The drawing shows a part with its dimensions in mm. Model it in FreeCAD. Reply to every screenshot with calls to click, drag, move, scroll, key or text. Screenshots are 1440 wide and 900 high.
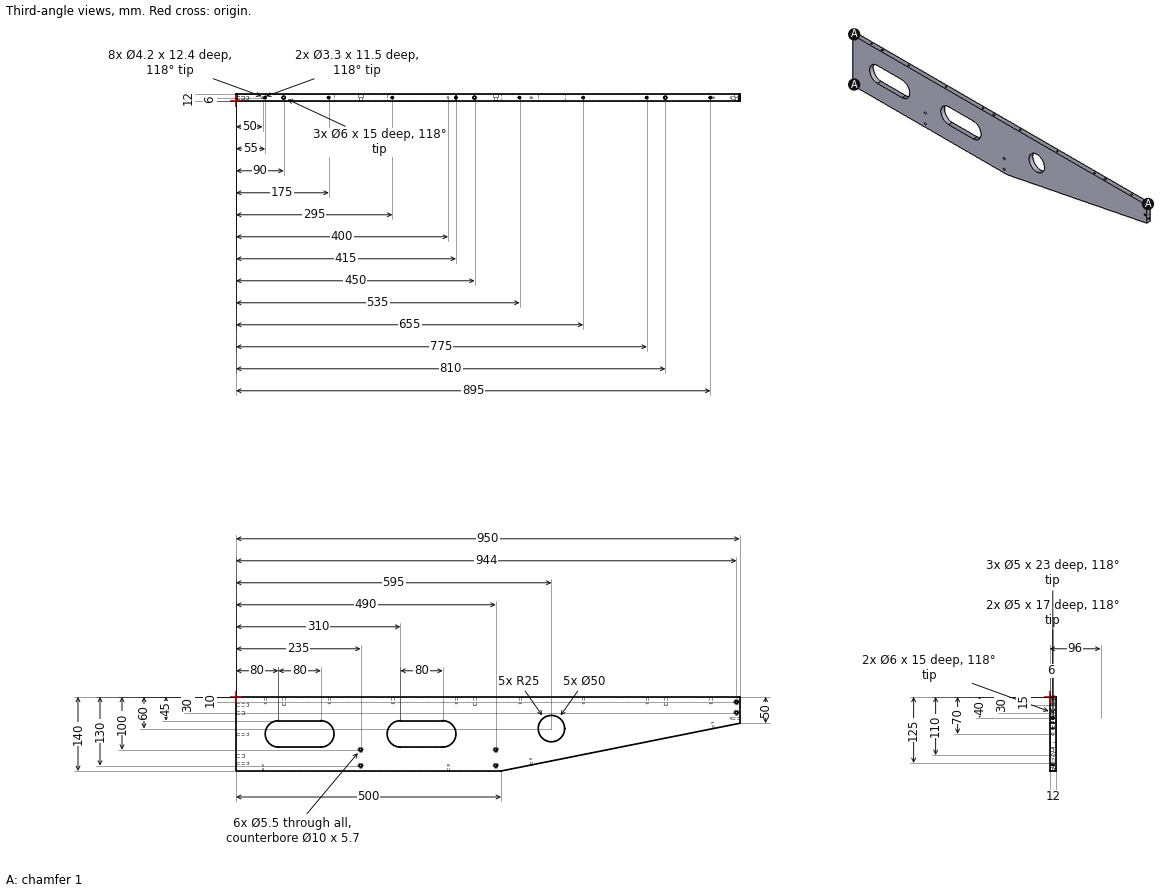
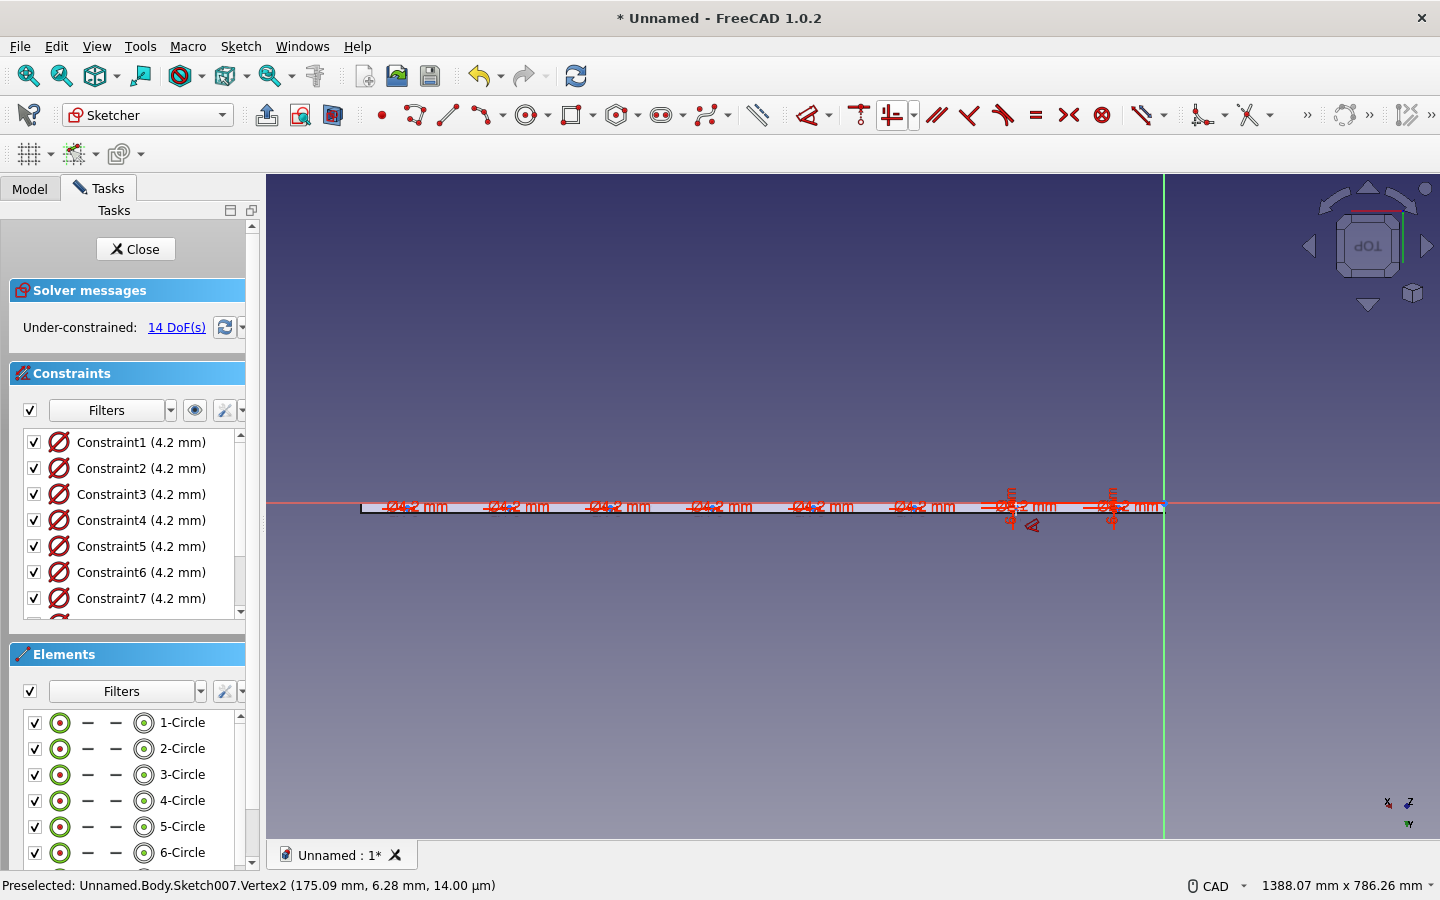
scroll(915, 509, up, 11)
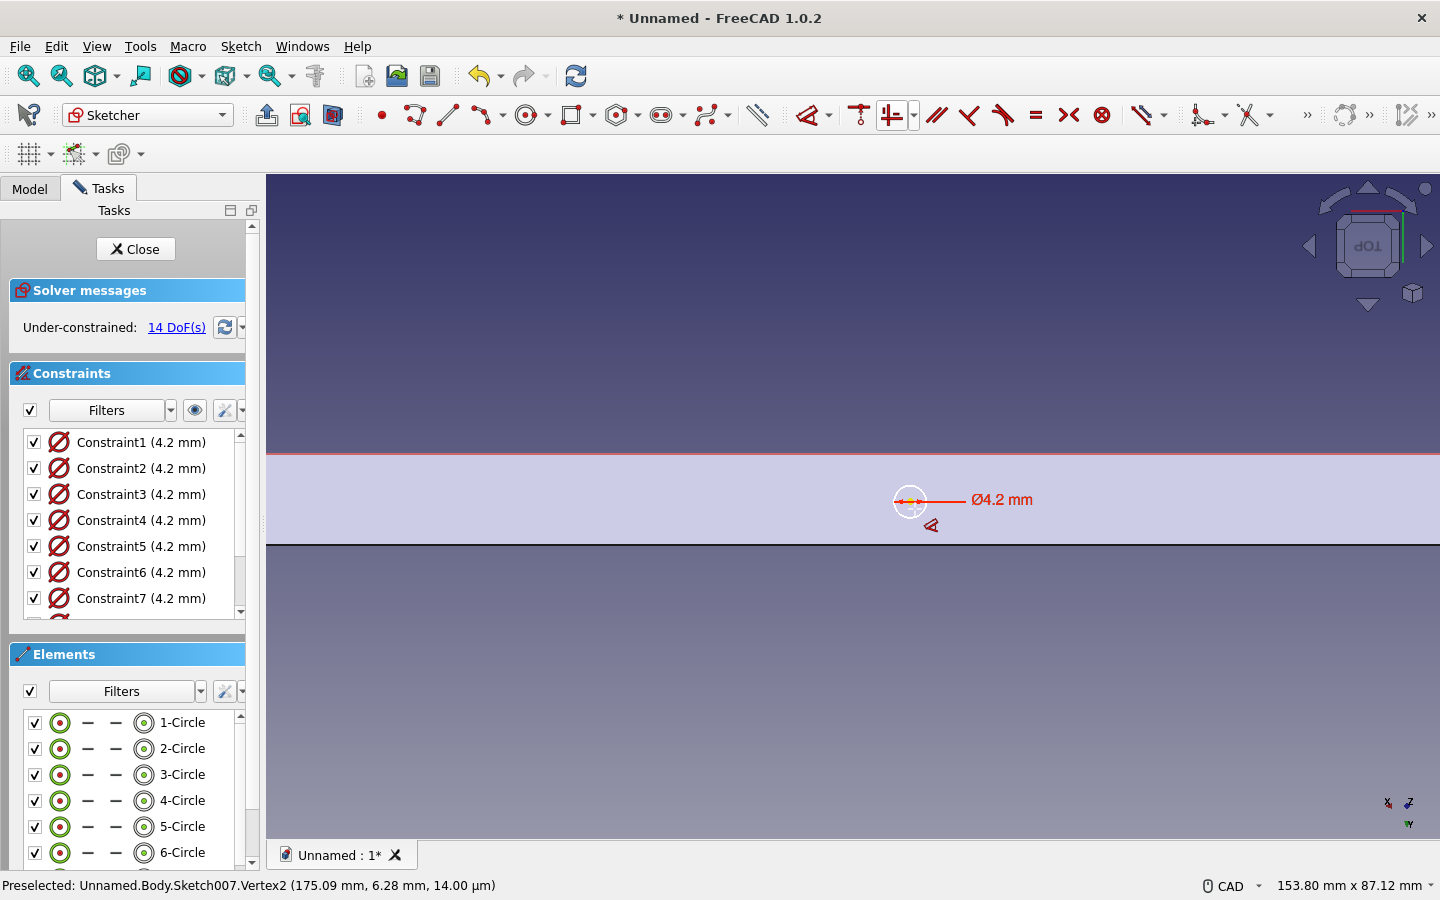
click(910, 502)
click(876, 478)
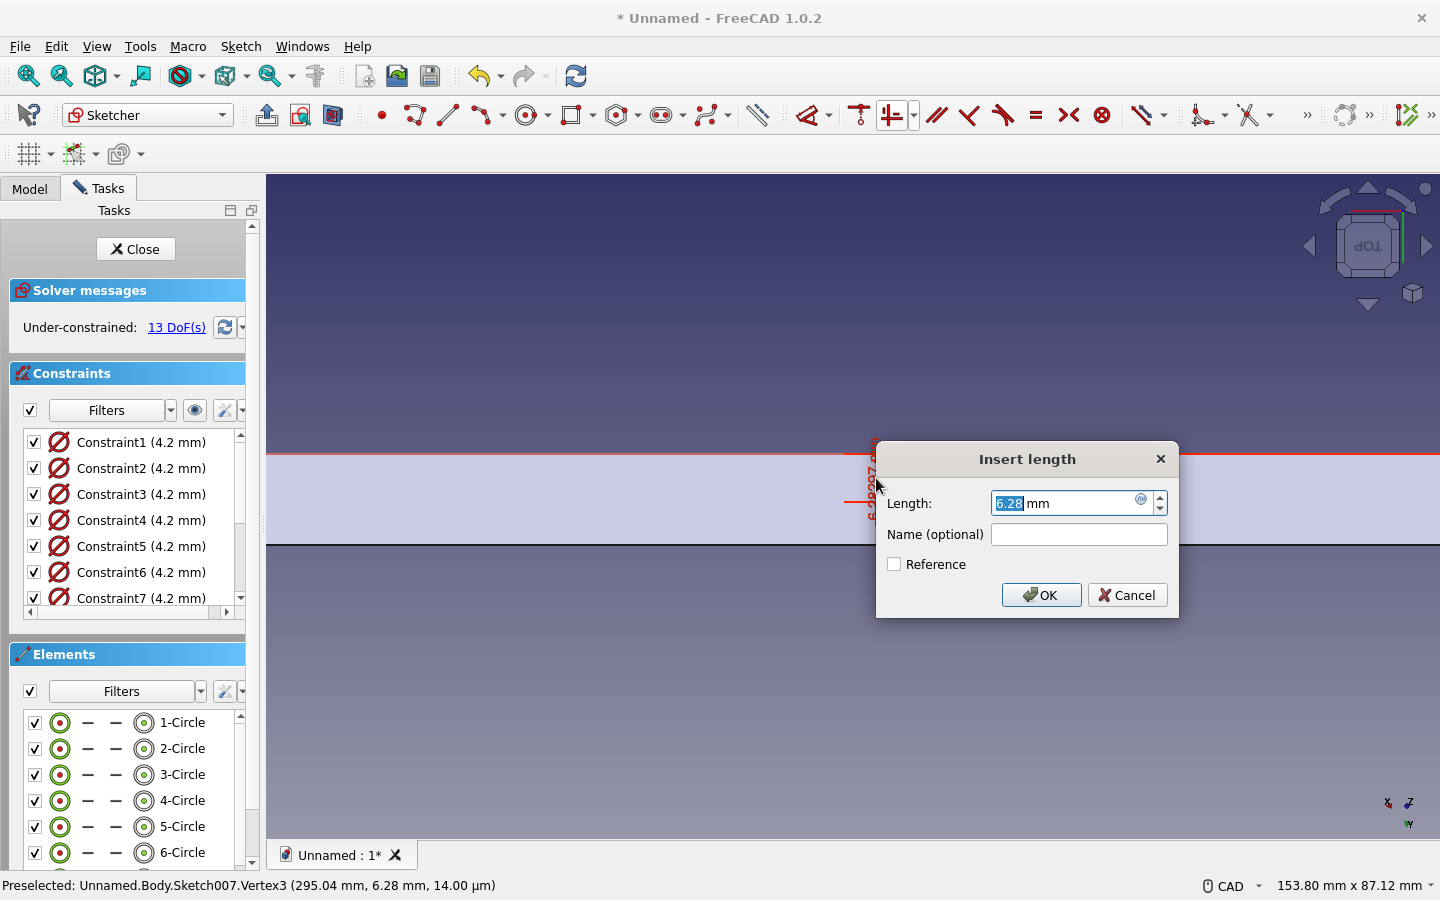
text(6)
key(Return)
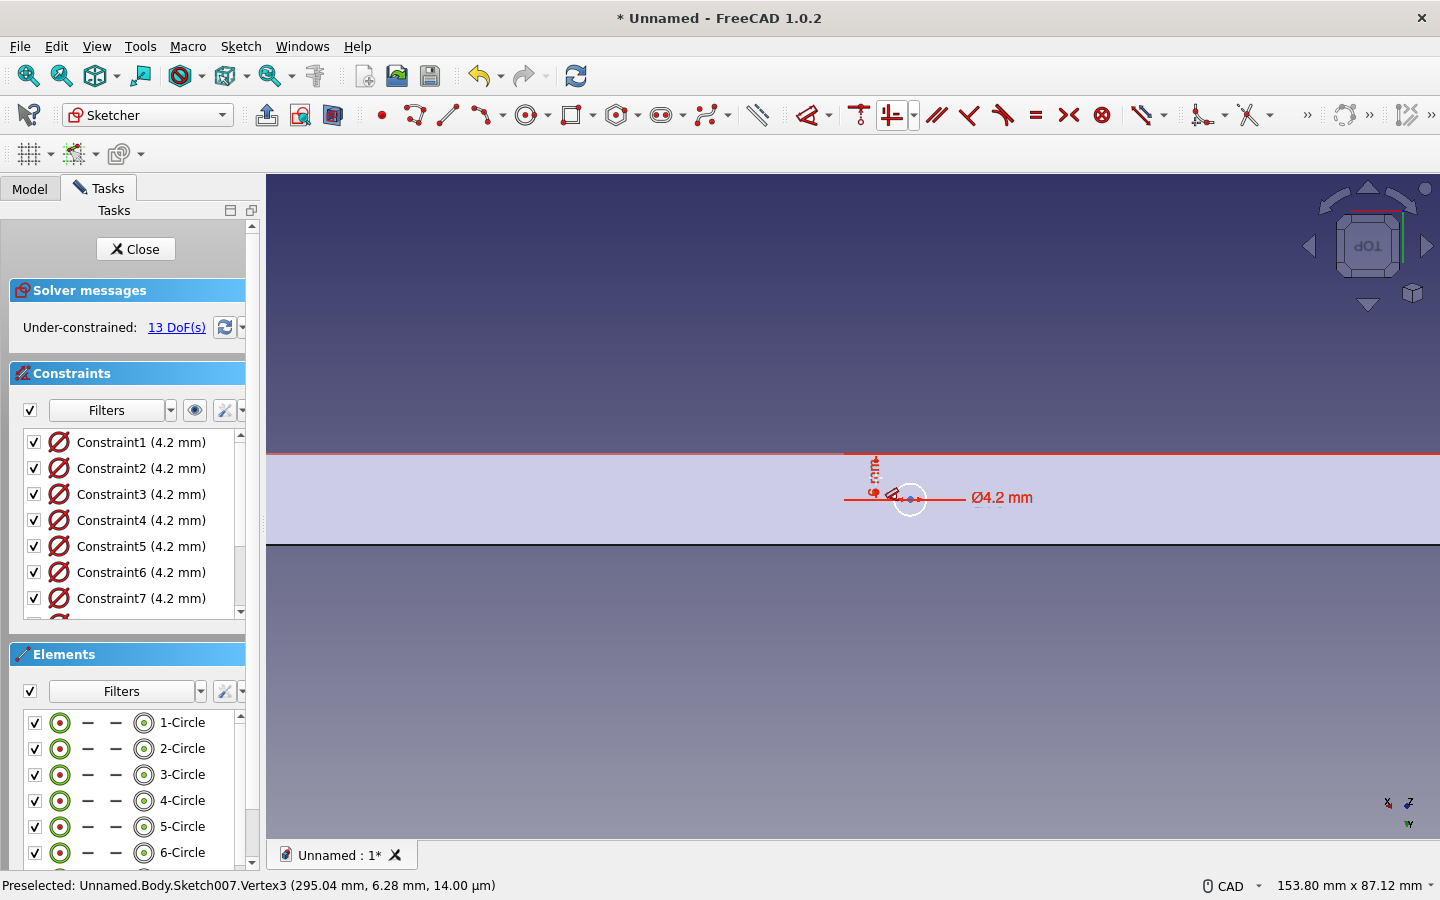
scroll(915, 509, down, 11)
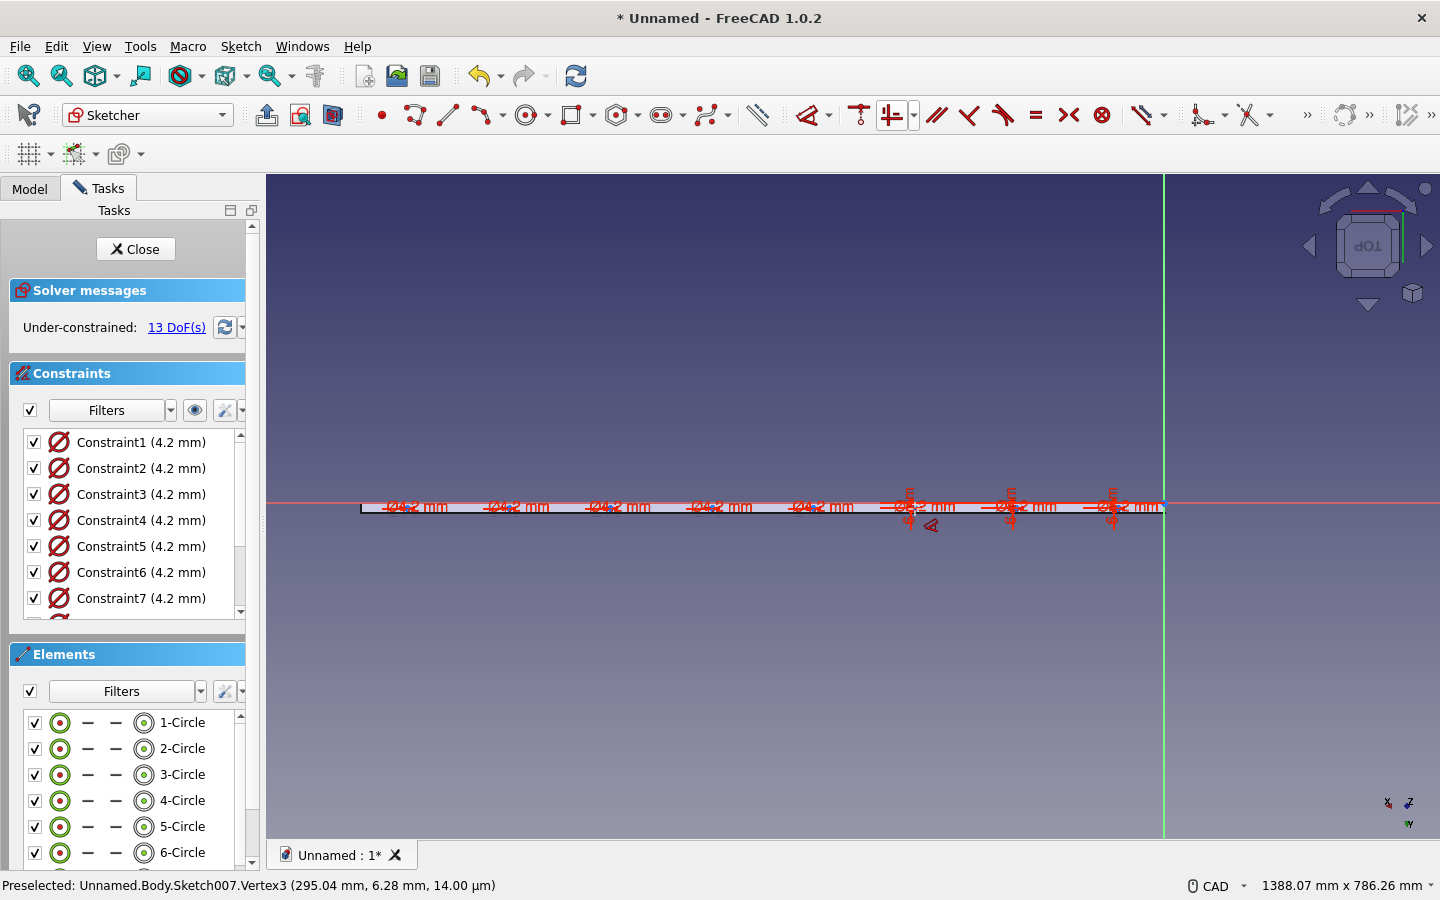
scroll(813, 509, up, 11)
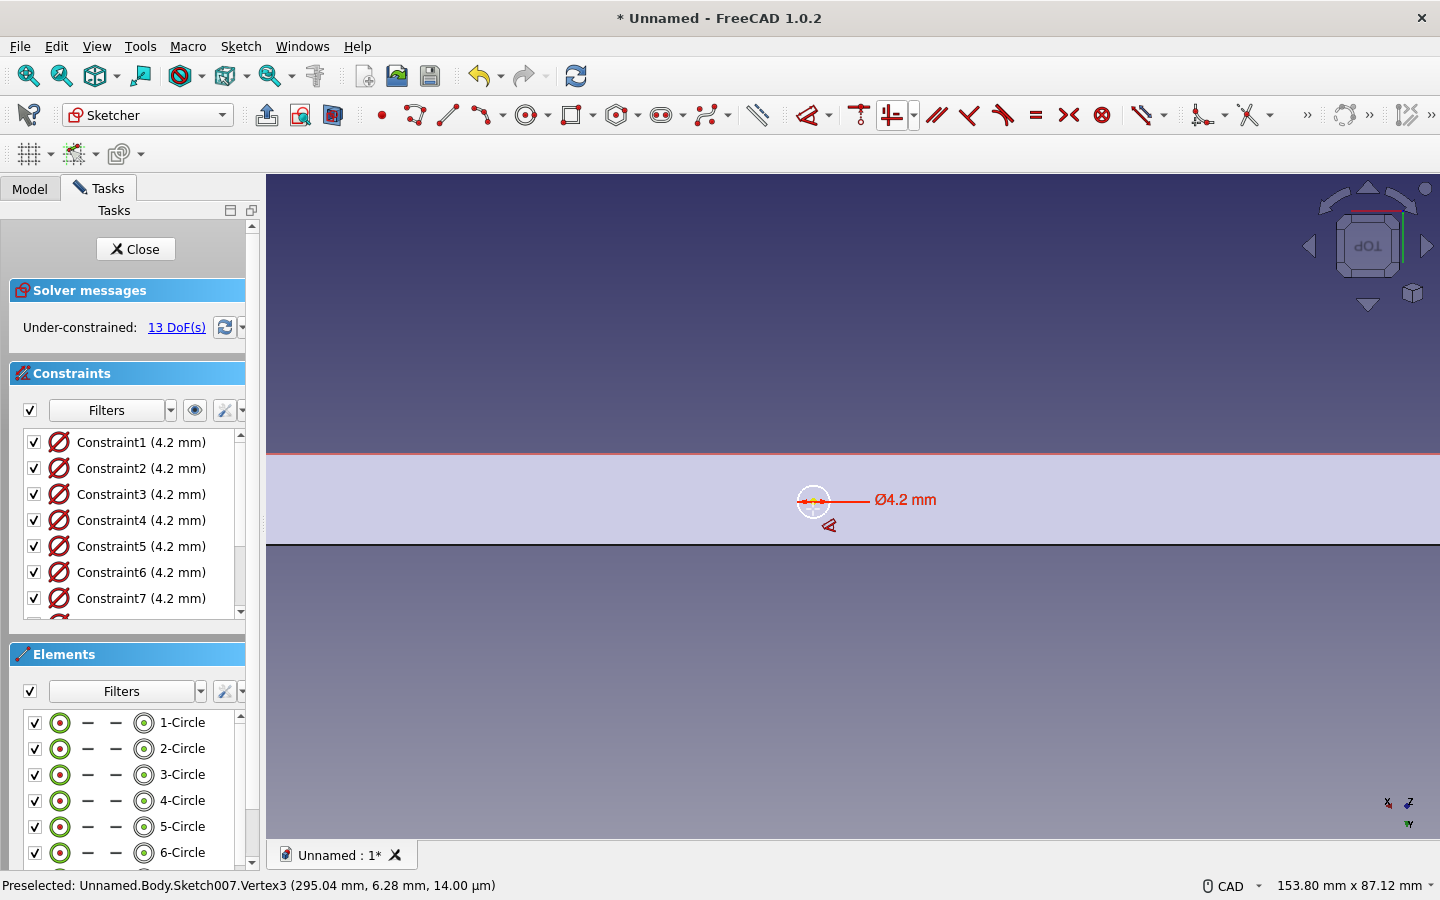
click(814, 502)
click(780, 478)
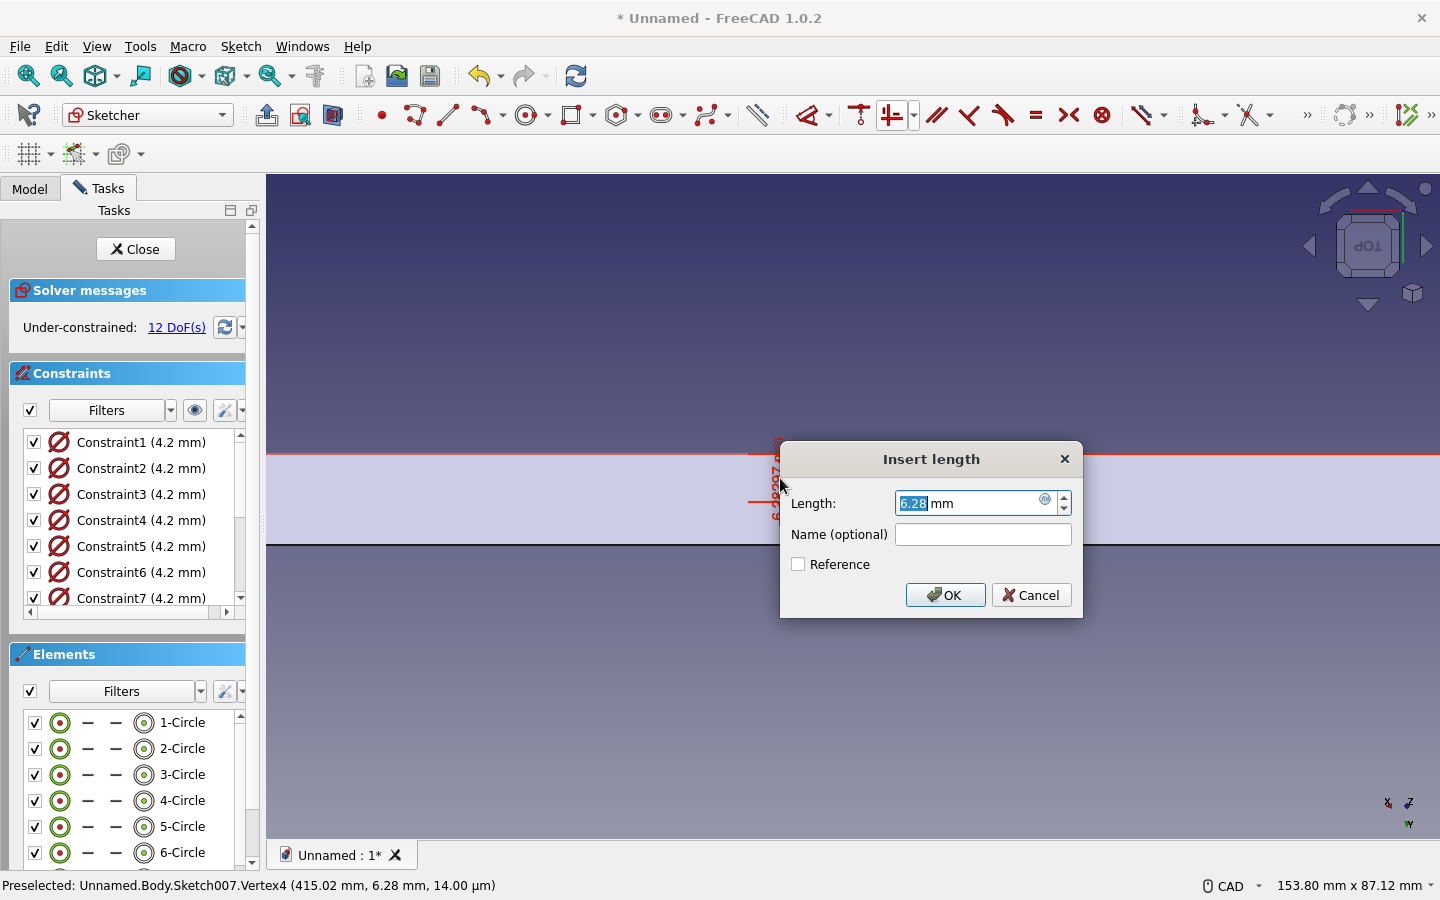
text(6)
key(Return)